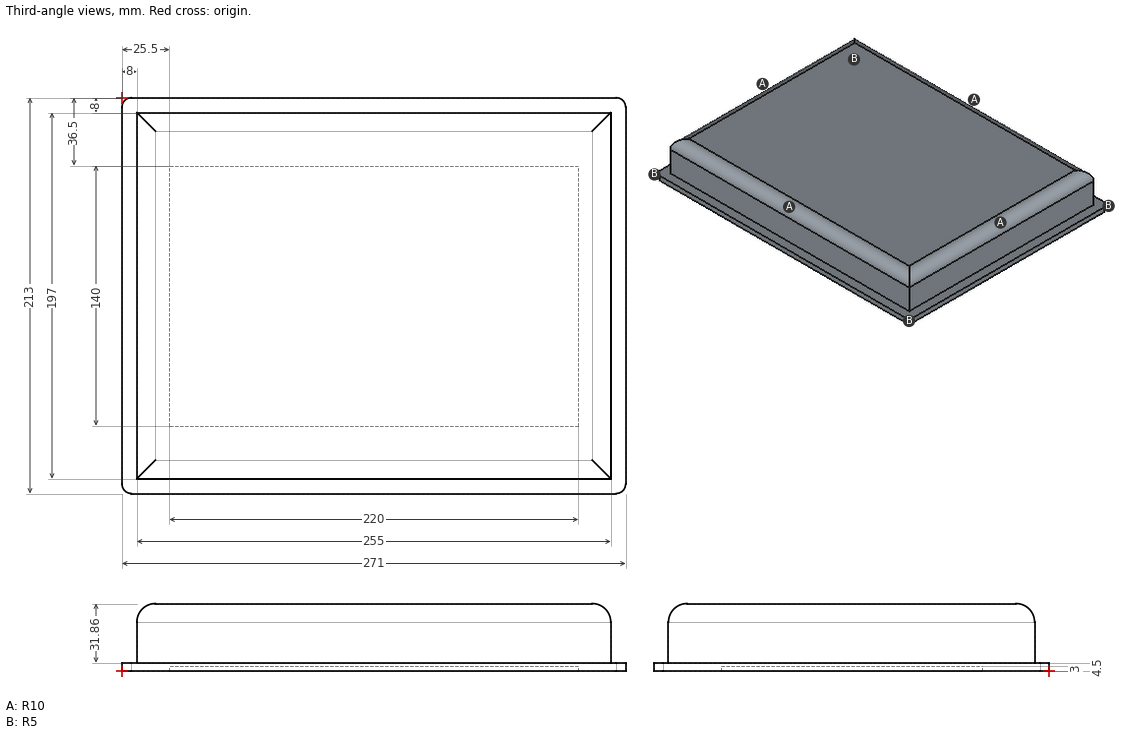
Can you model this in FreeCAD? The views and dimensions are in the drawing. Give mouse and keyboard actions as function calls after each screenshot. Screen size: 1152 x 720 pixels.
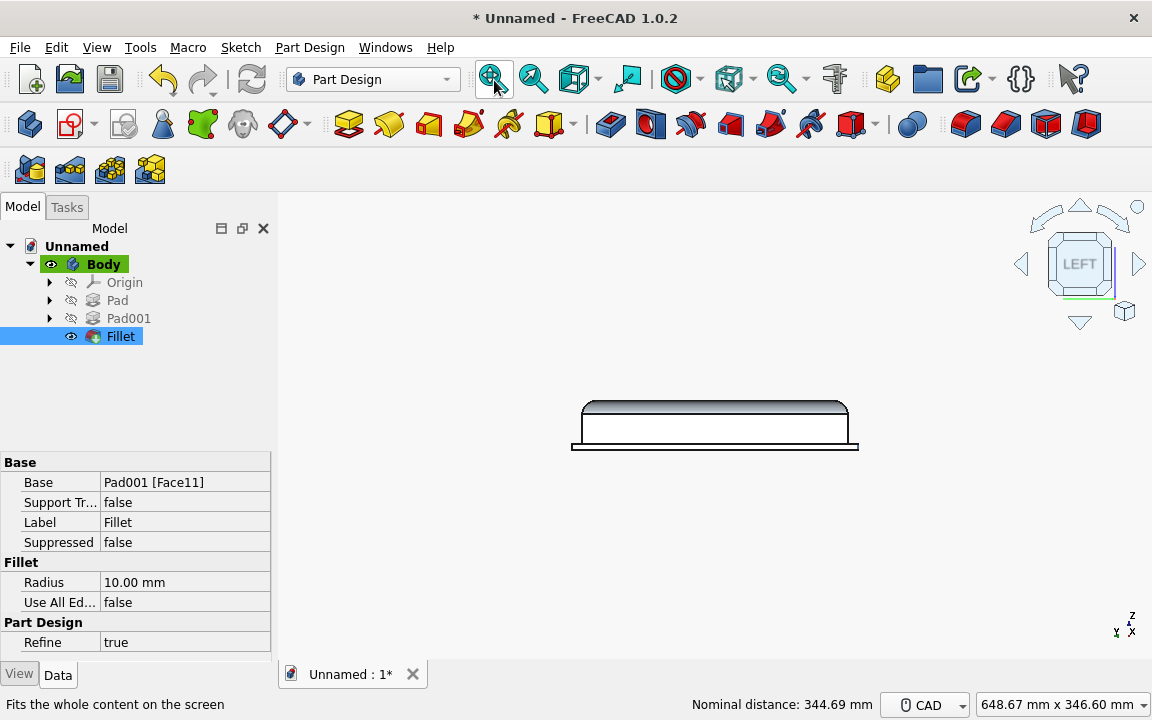
scroll(572, 446, up, 10)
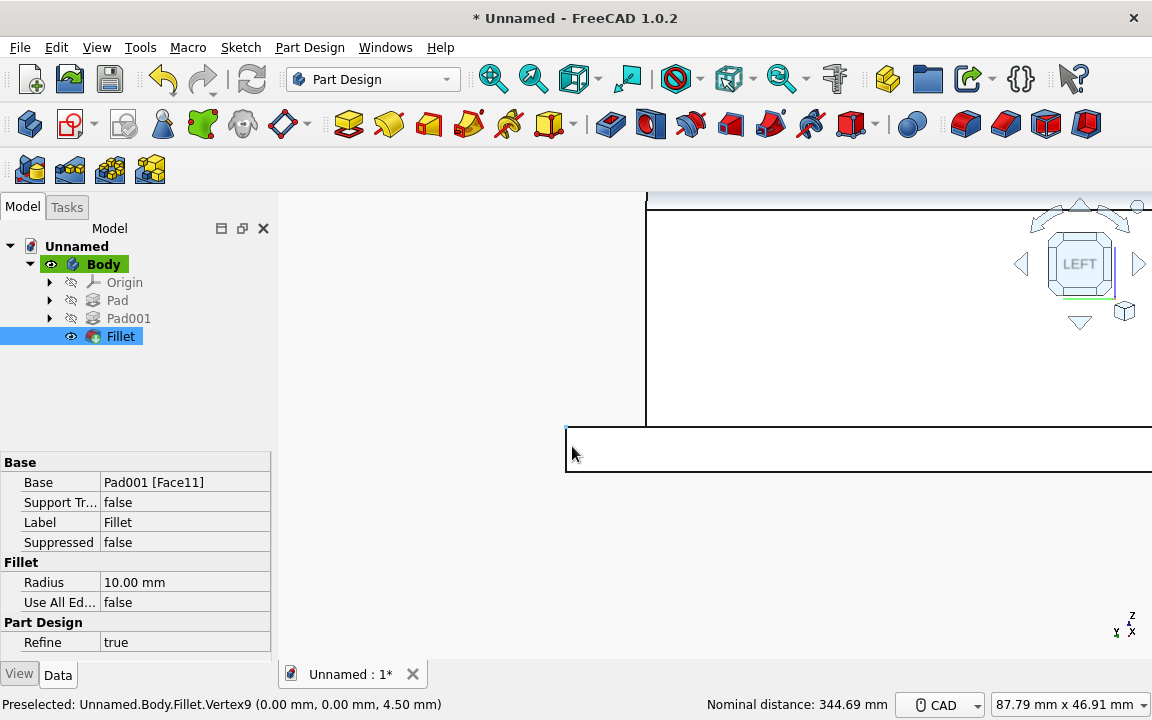
click(566, 449, ctrl)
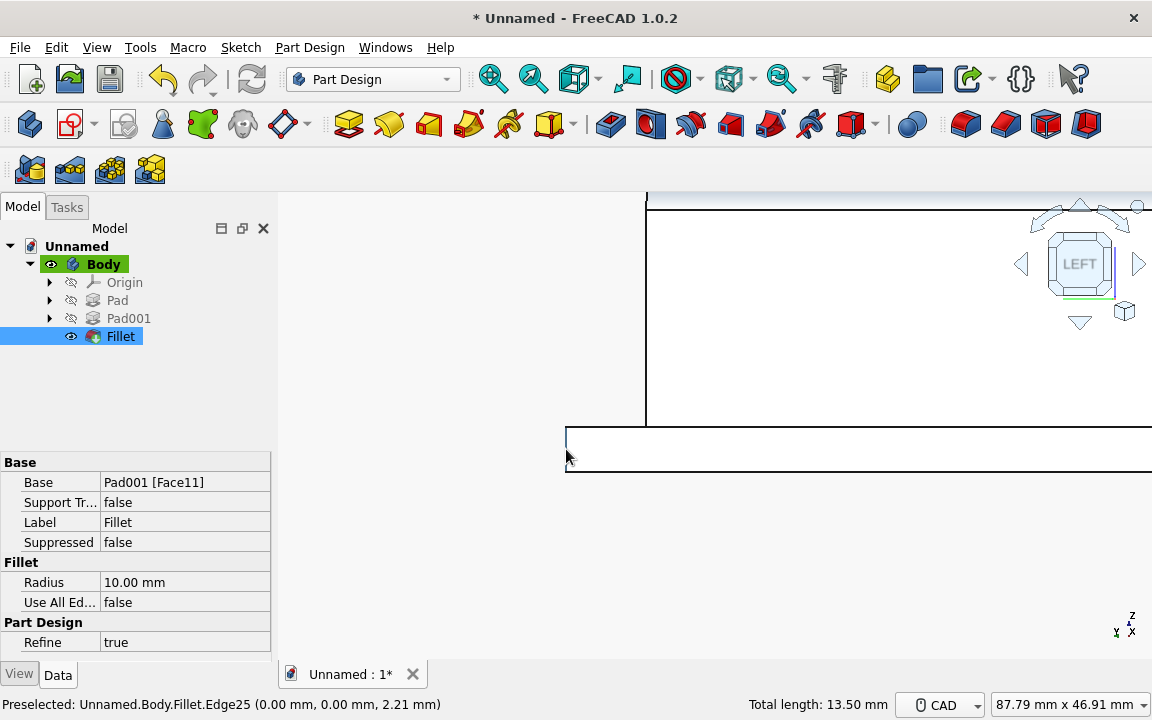
click(494, 80)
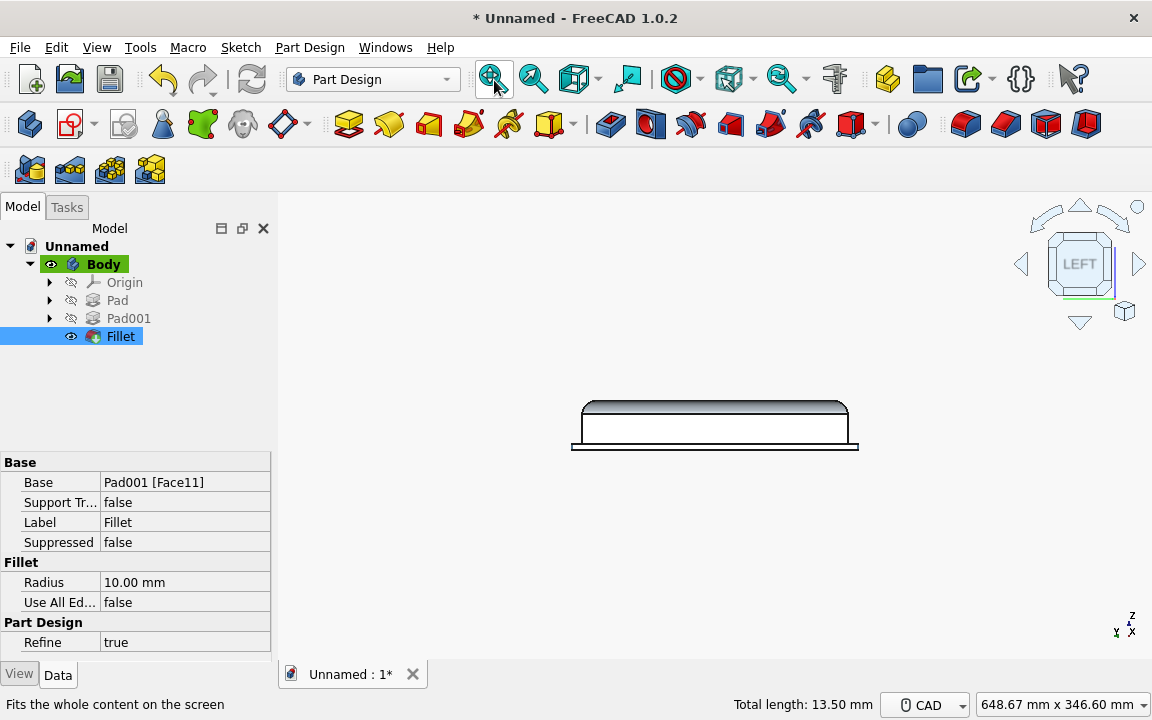
key(v)
key(3)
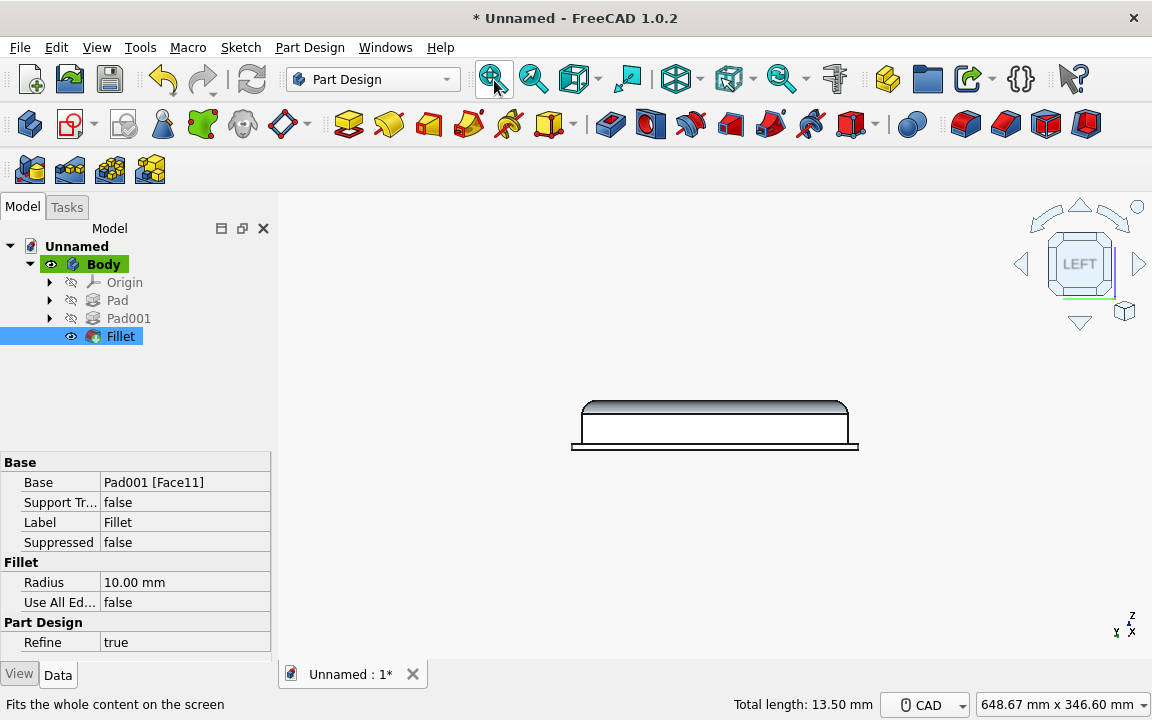
key(0)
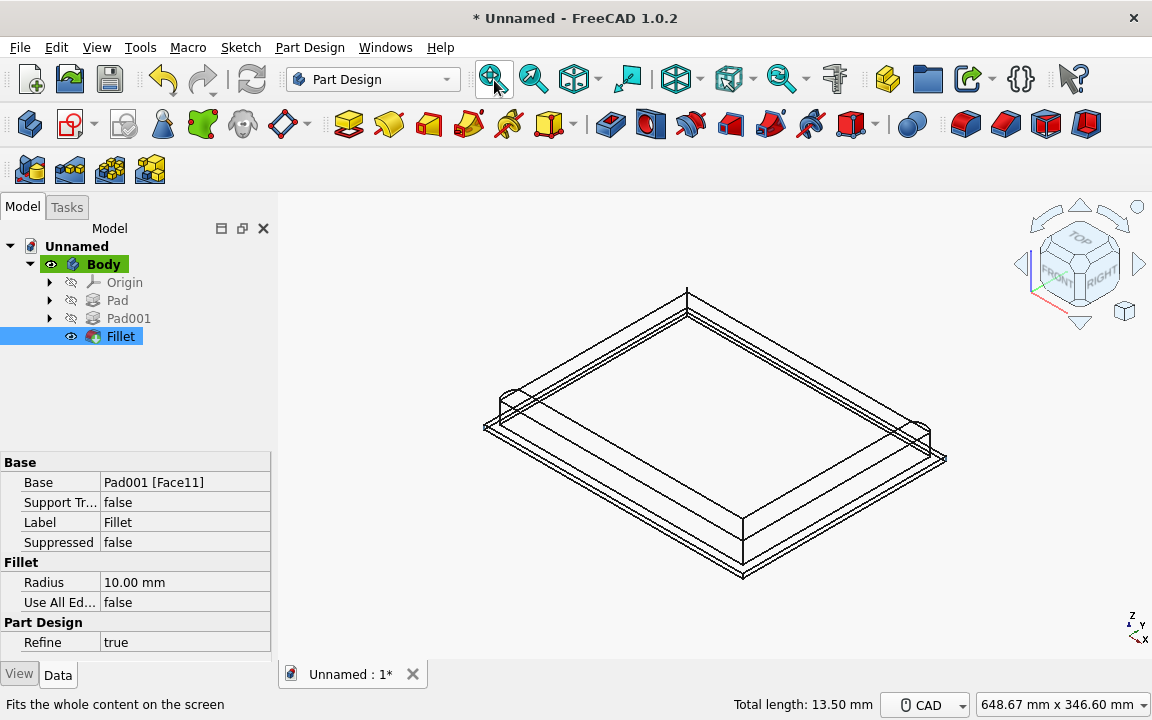
scroll(743, 575, up, 10)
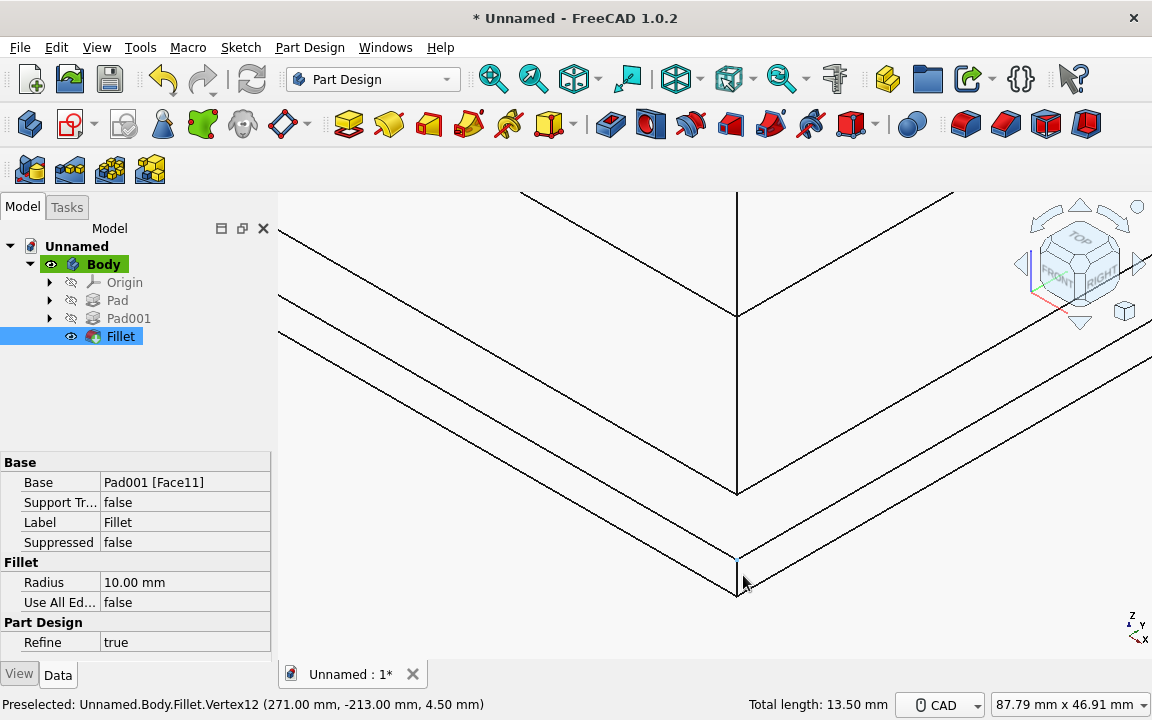
click(737, 577, ctrl)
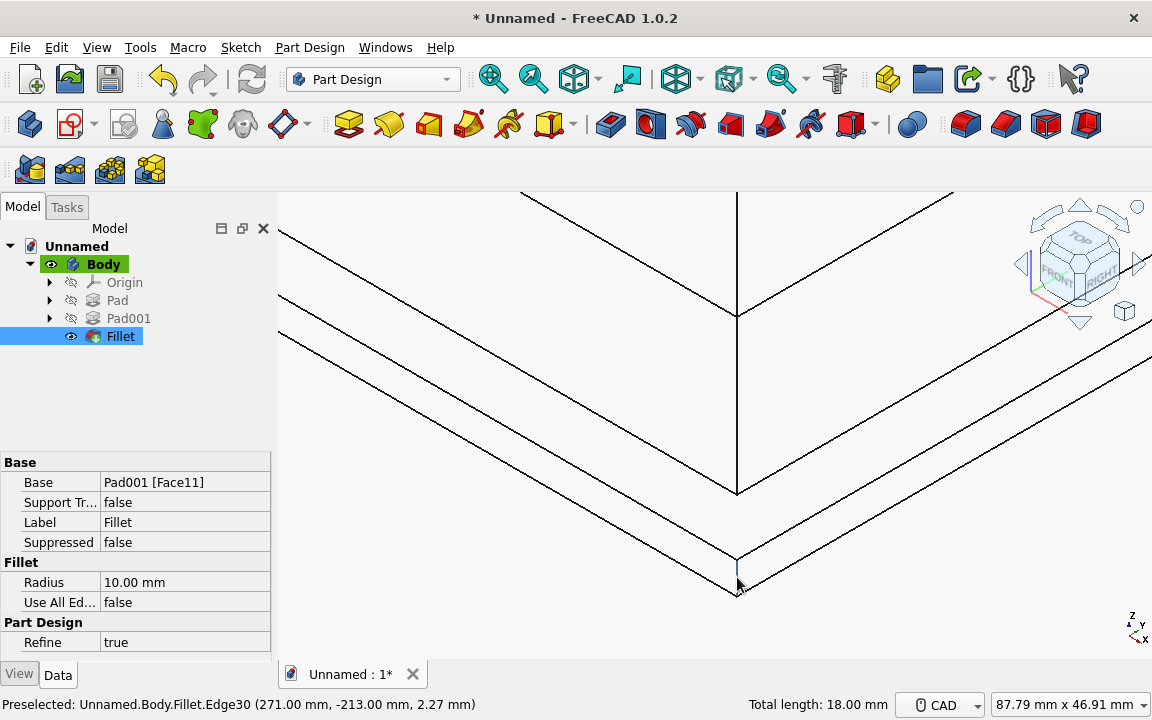
key(v)
key(1)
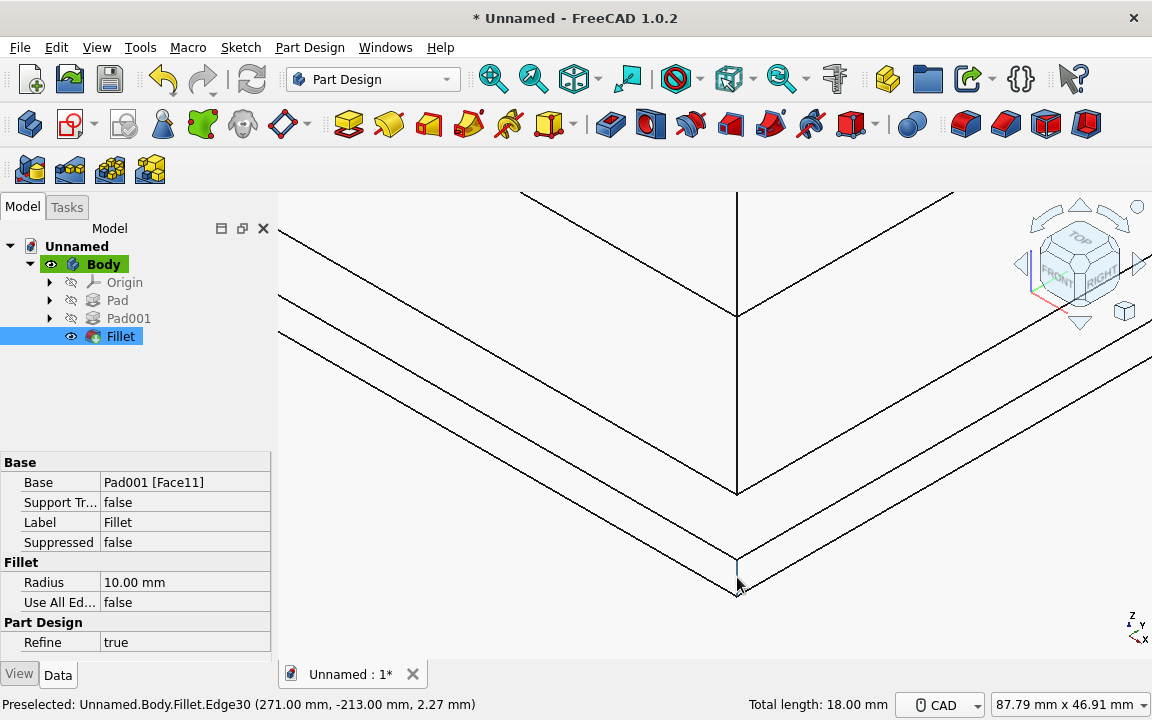
click(966, 124)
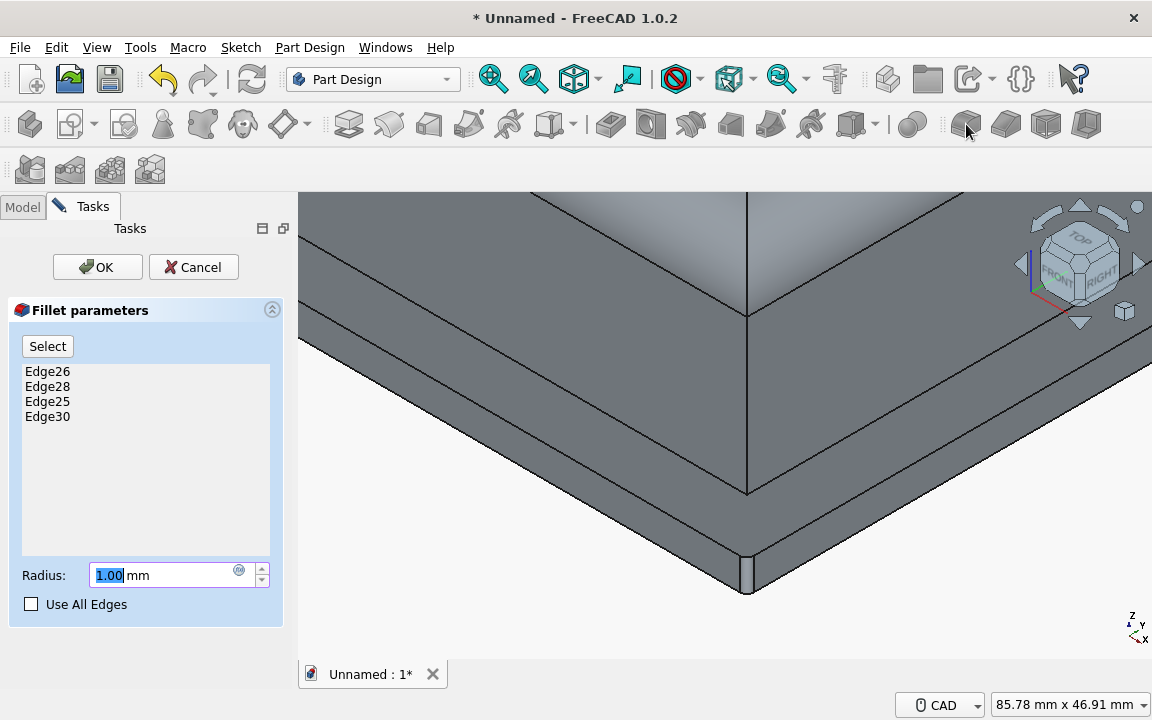
text(5)
key(Tab)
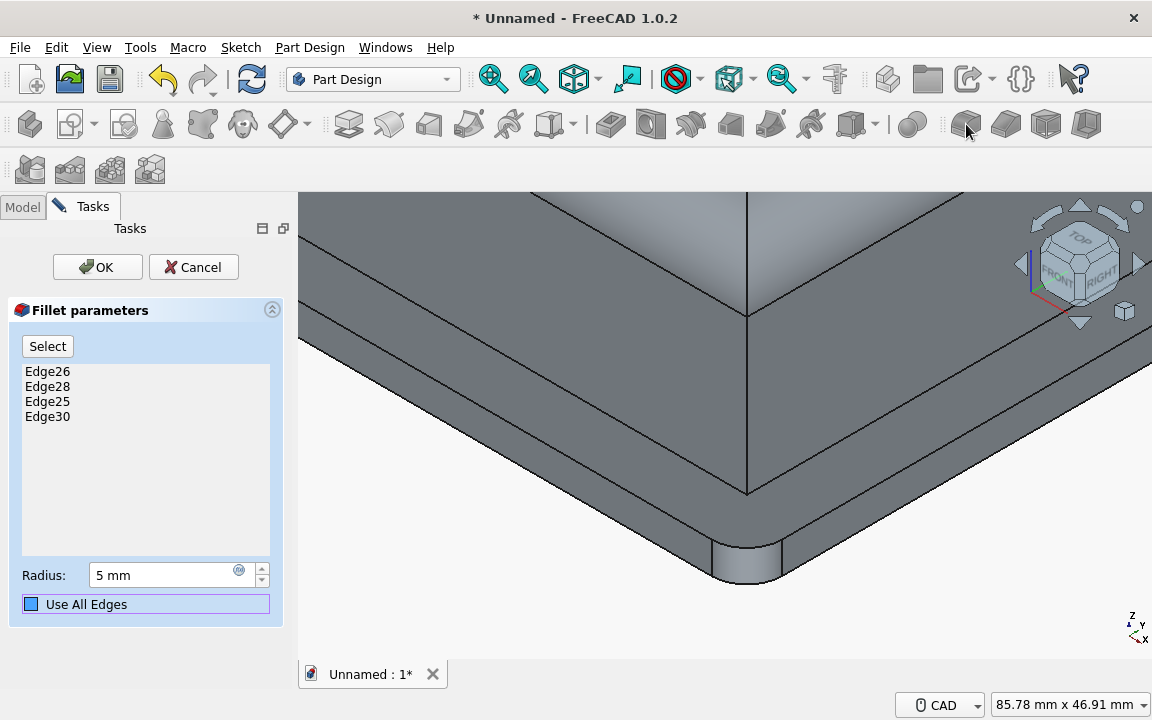
click(98, 267)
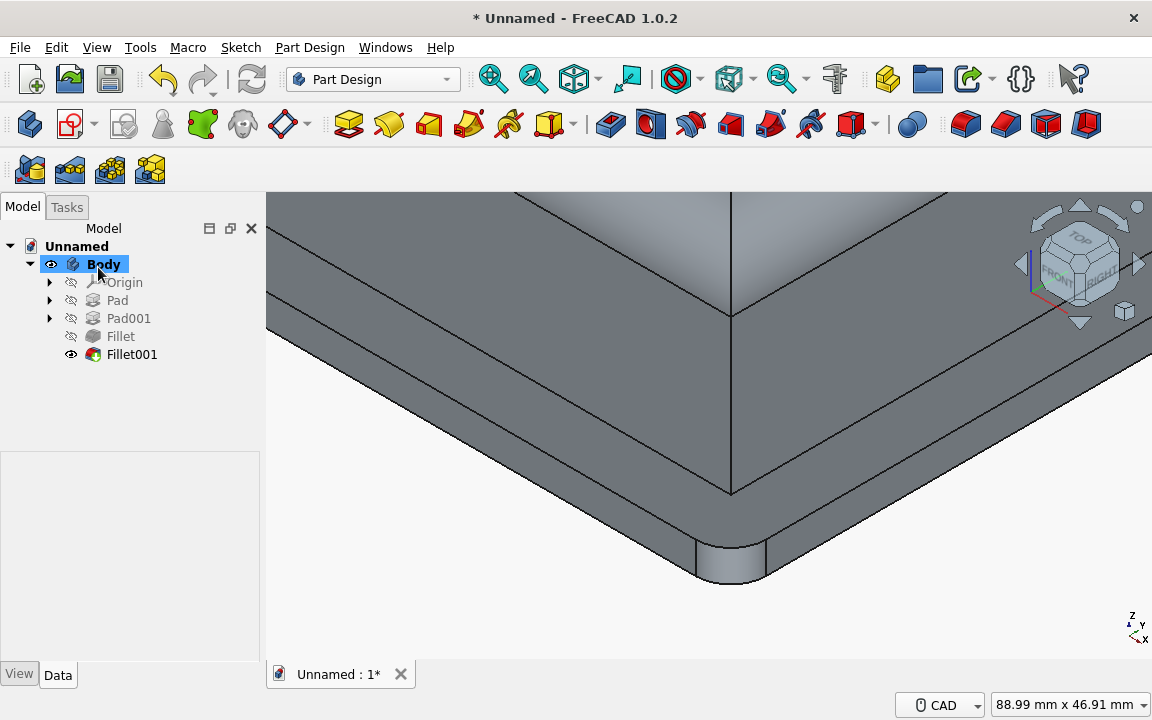
click(494, 80)